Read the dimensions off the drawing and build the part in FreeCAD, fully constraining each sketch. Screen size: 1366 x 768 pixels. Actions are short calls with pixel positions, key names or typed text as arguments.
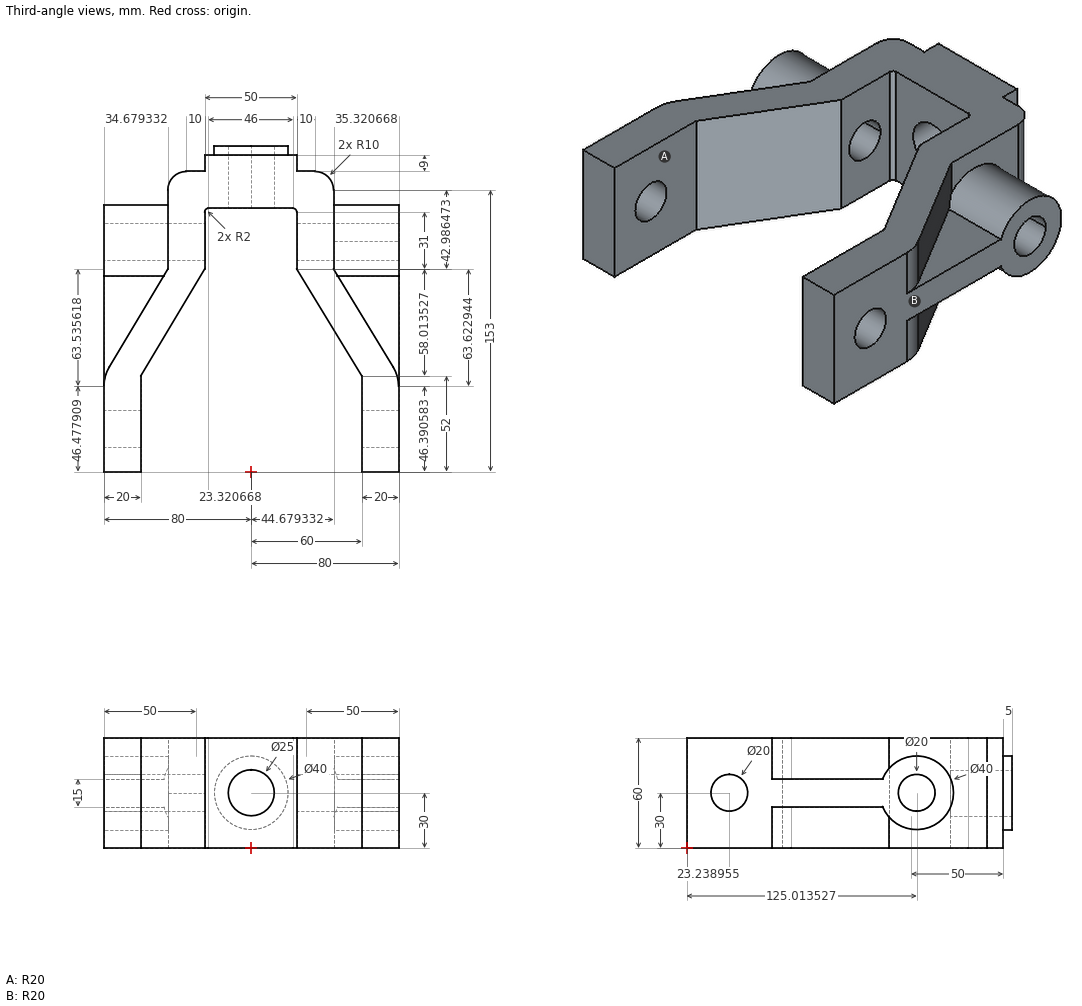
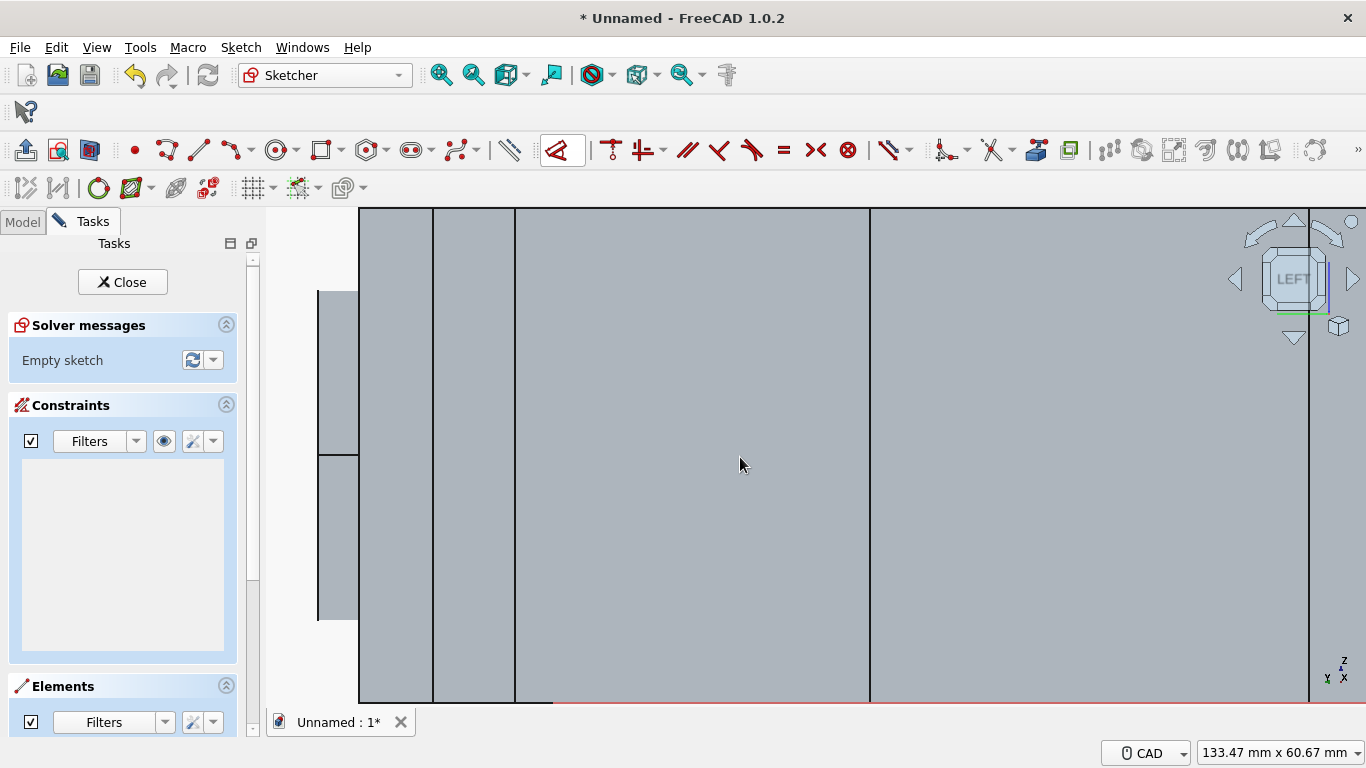
key(g)
key(c)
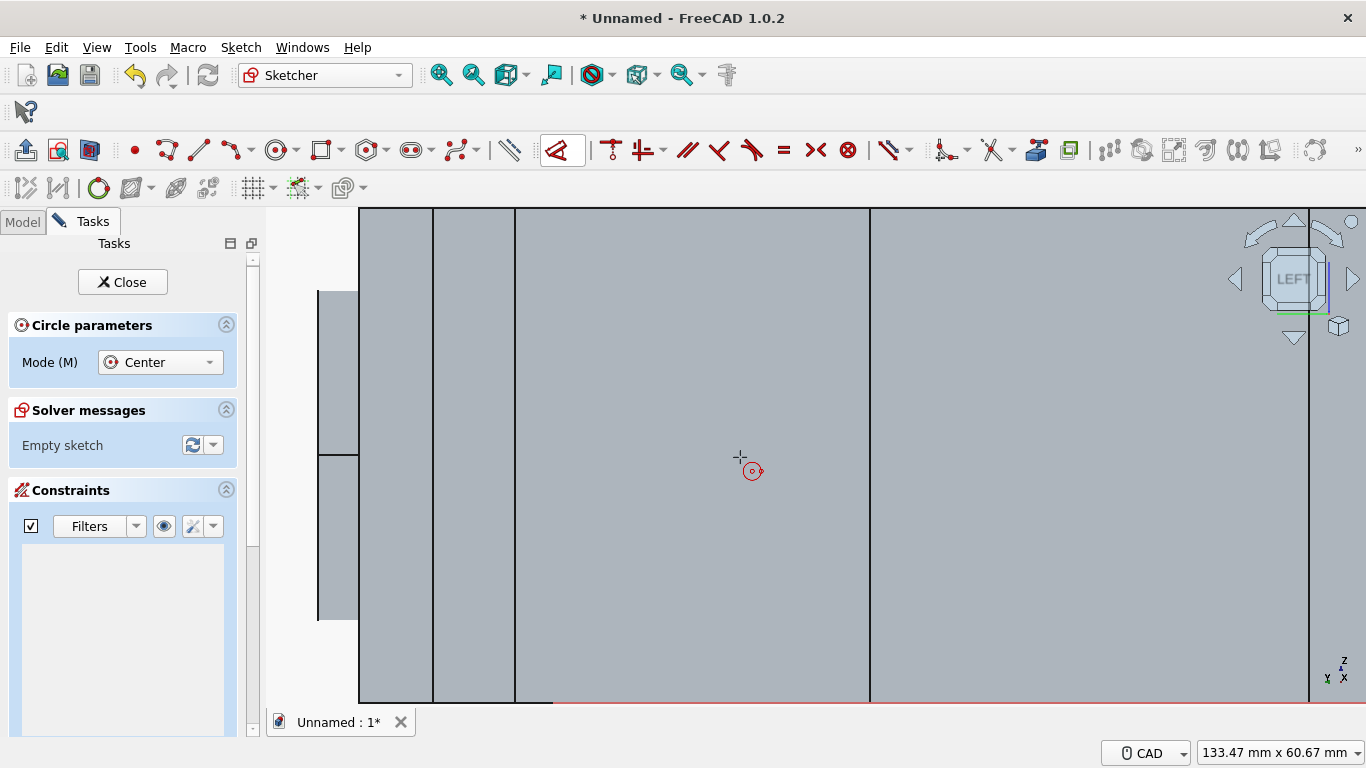
click(746, 455)
click(863, 339)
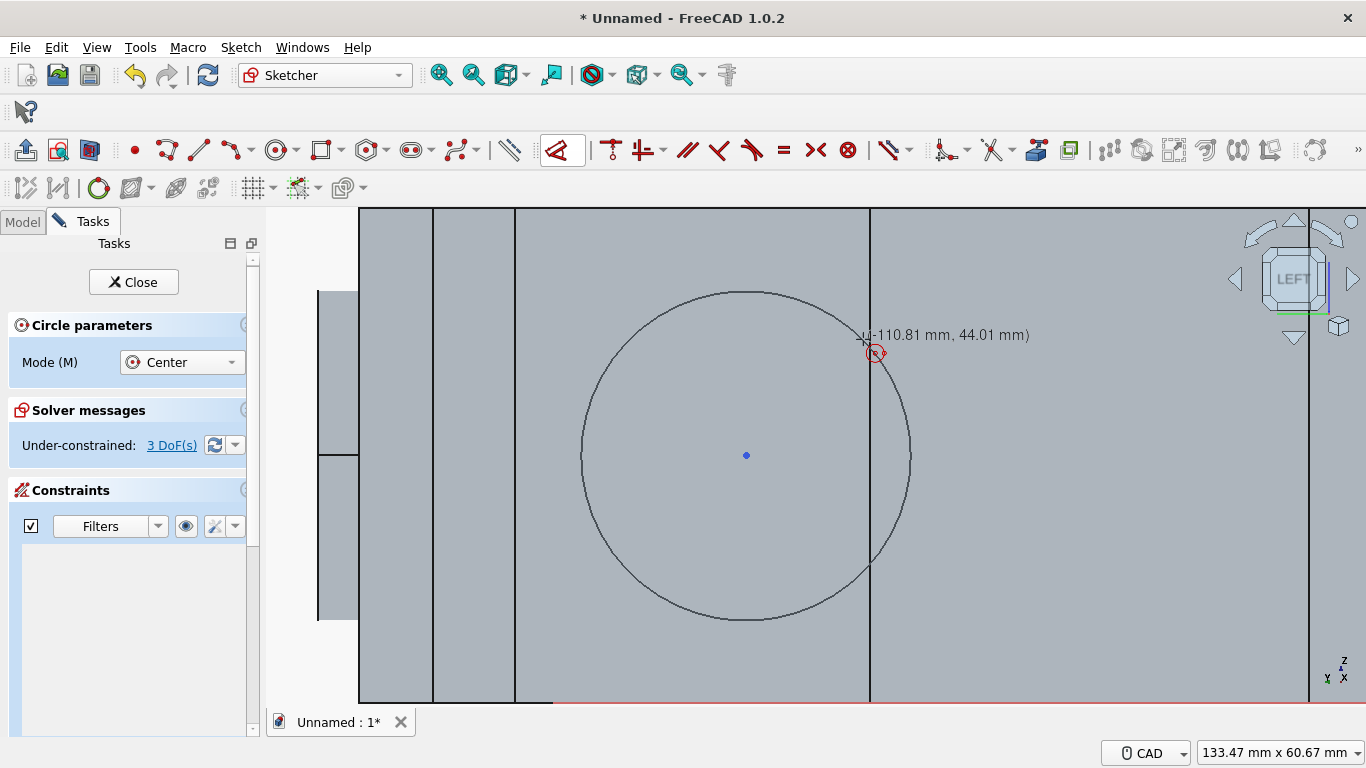
click(746, 456)
click(804, 397)
key(Escape)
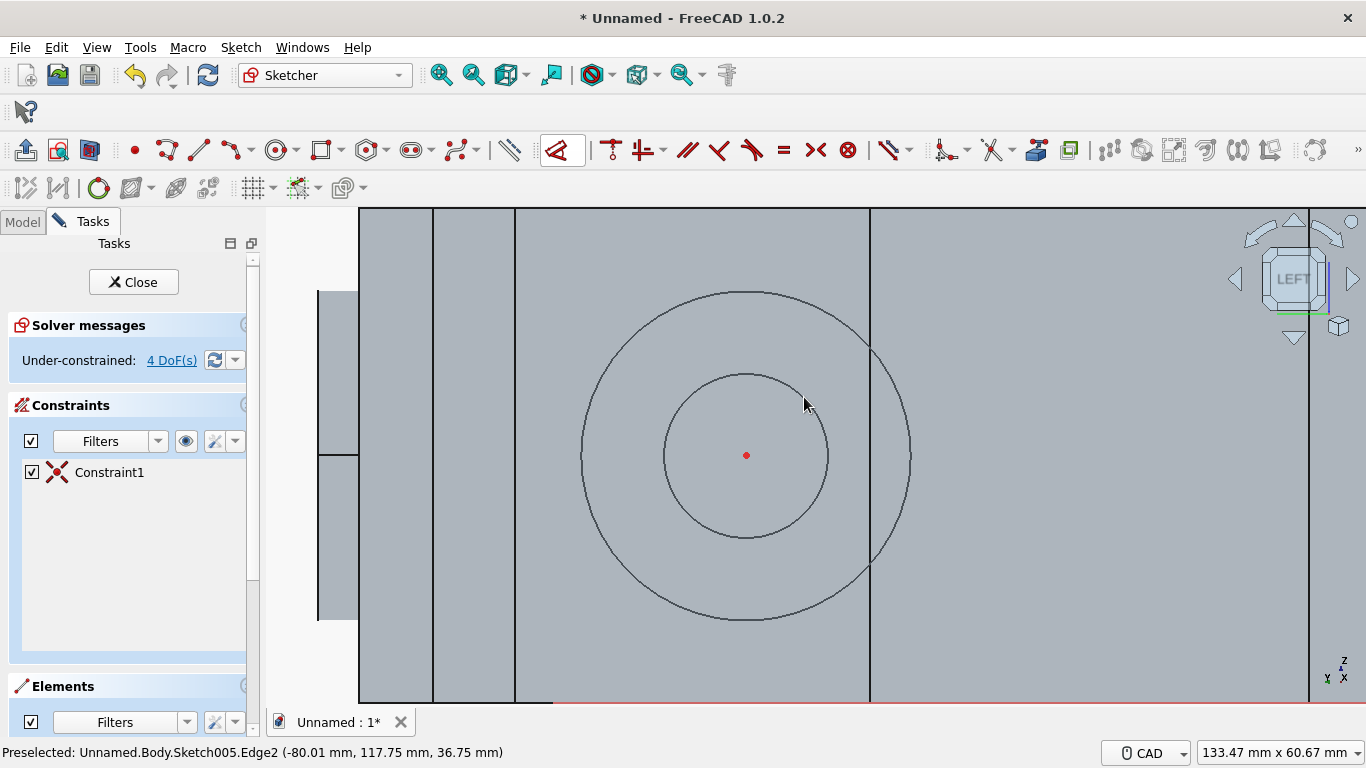
click(862, 339)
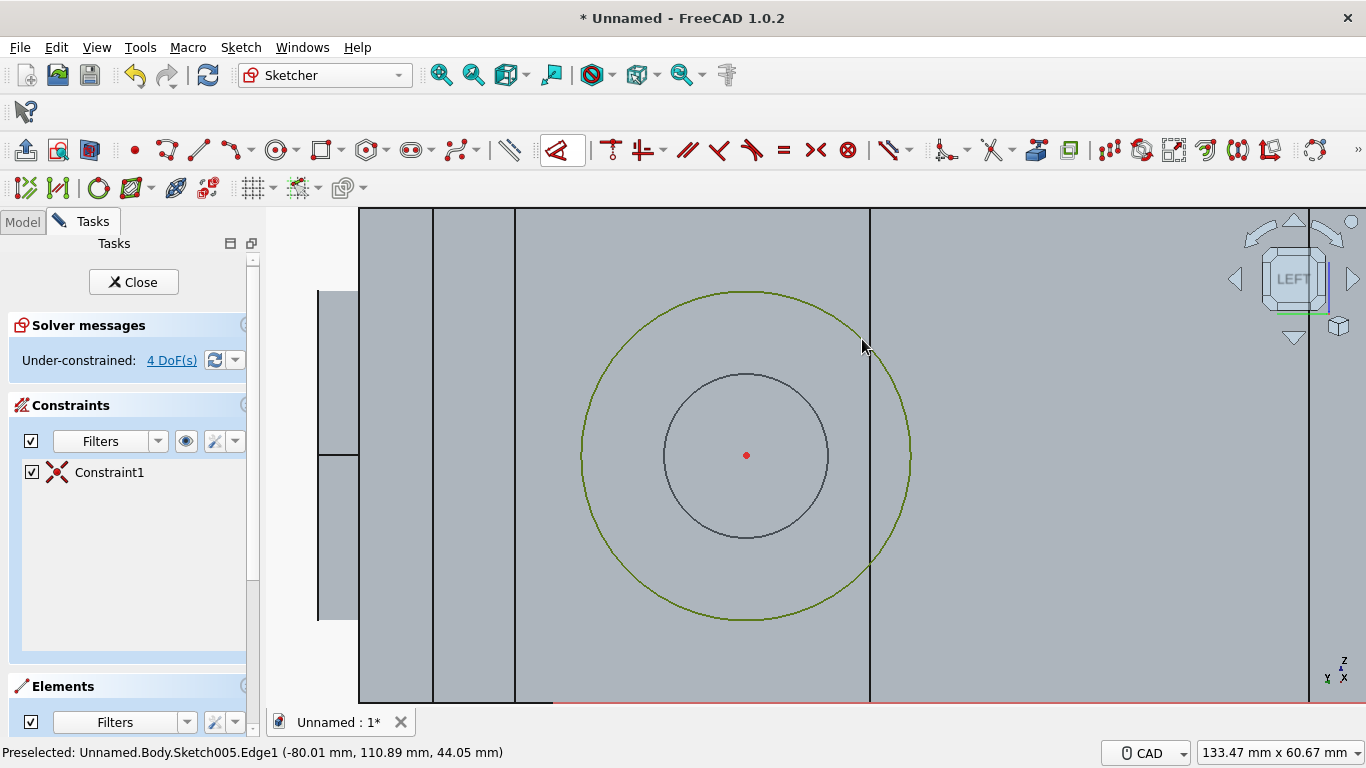
key(k)
key(o)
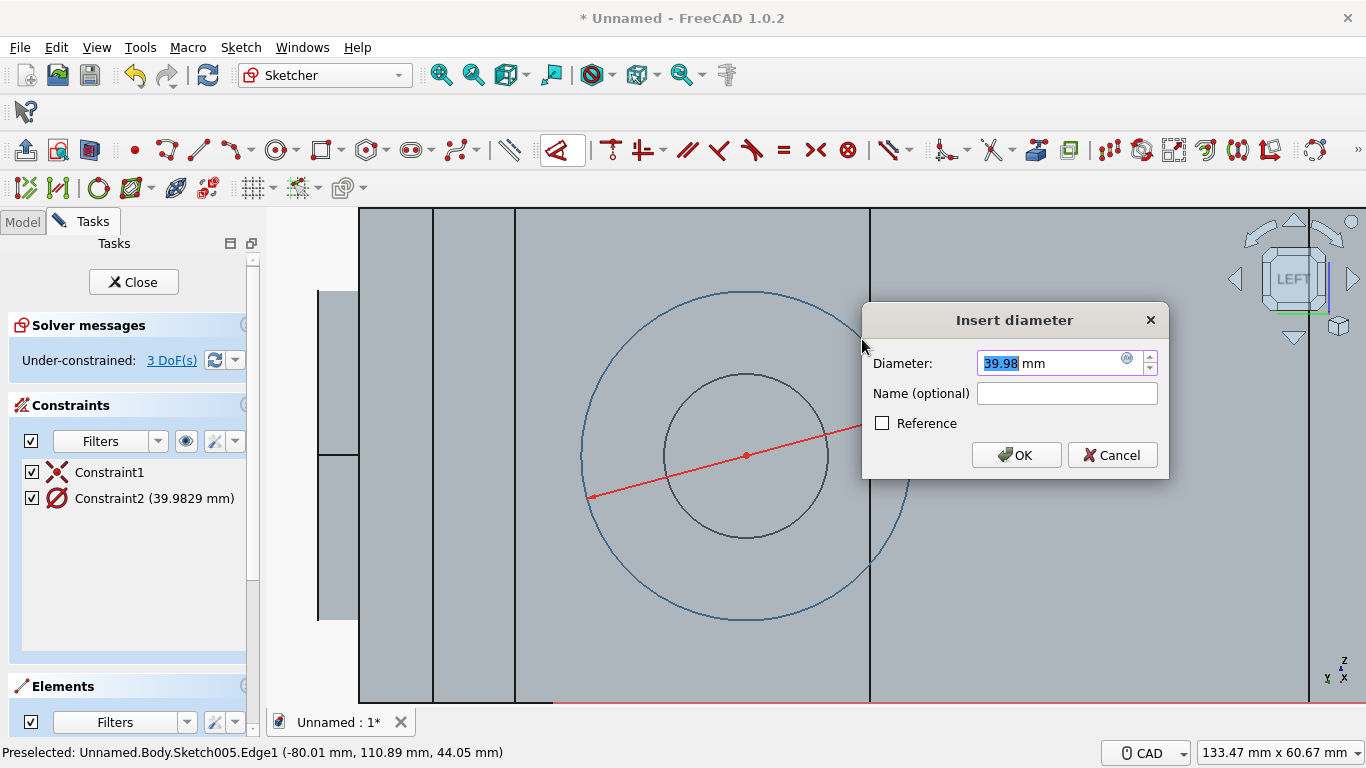
text(40)
key(Return)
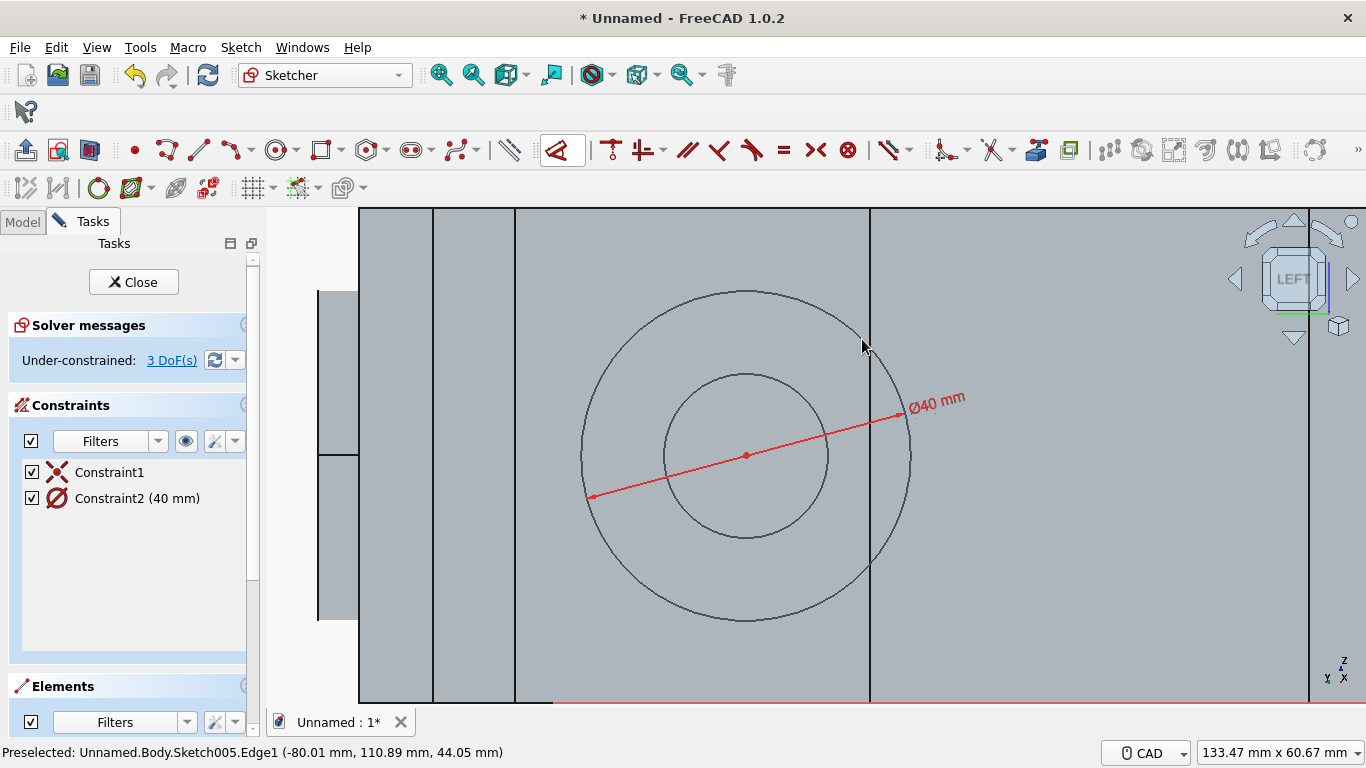
click(804, 398)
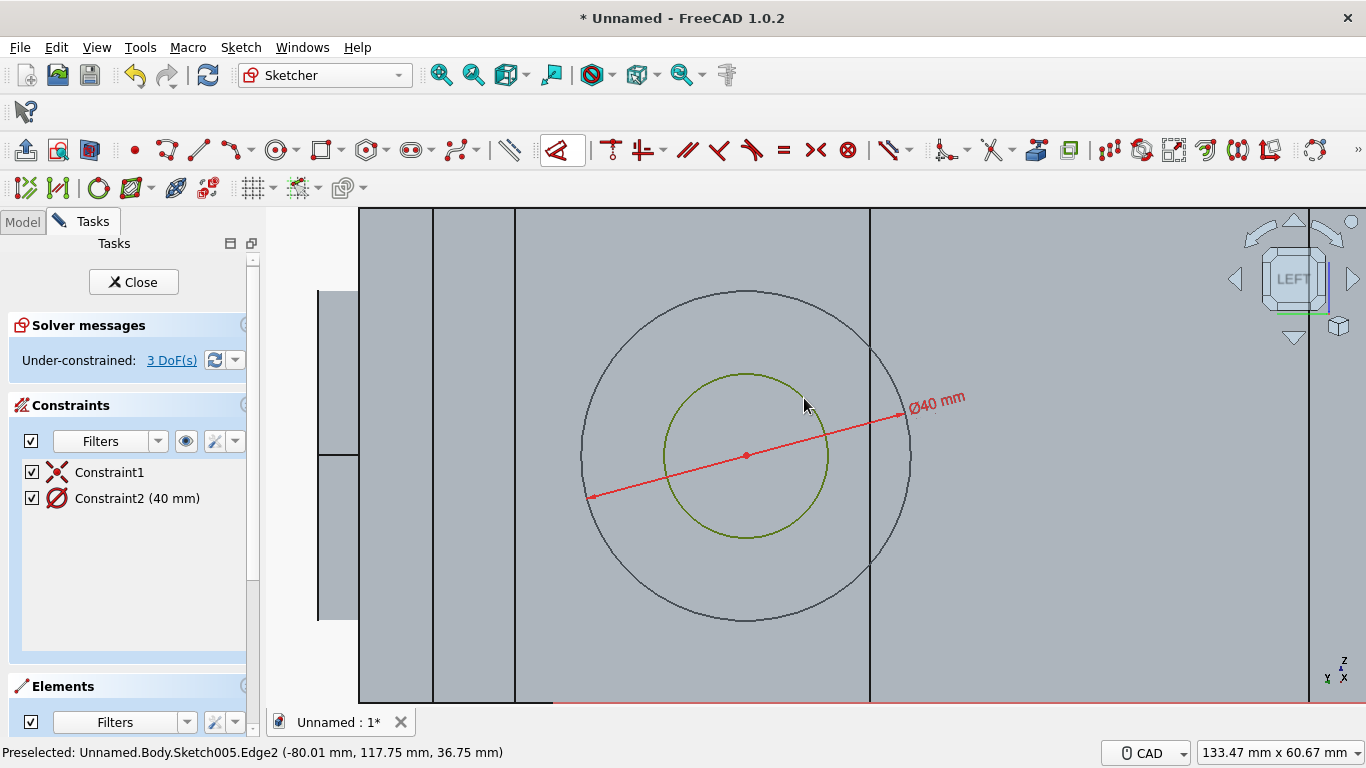
key(k)
key(o)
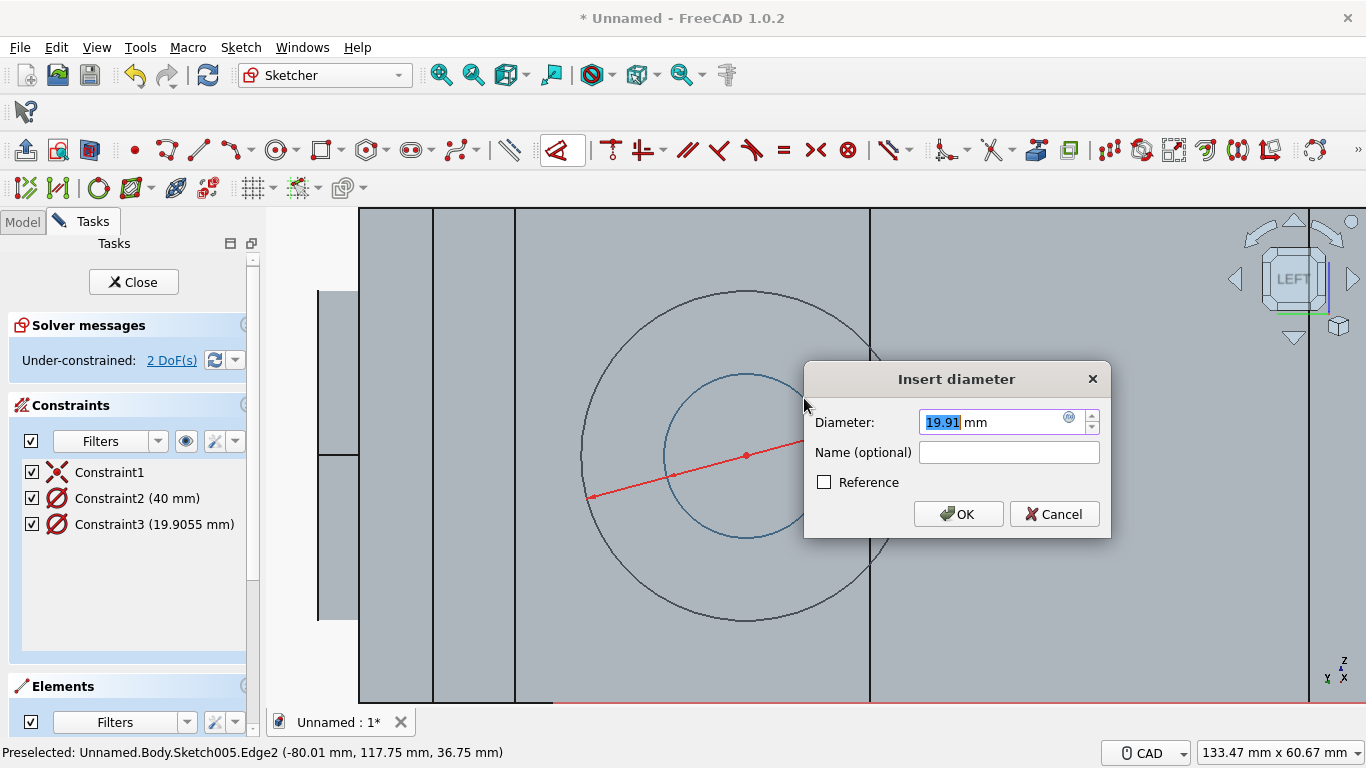
text(20)
key(Return)